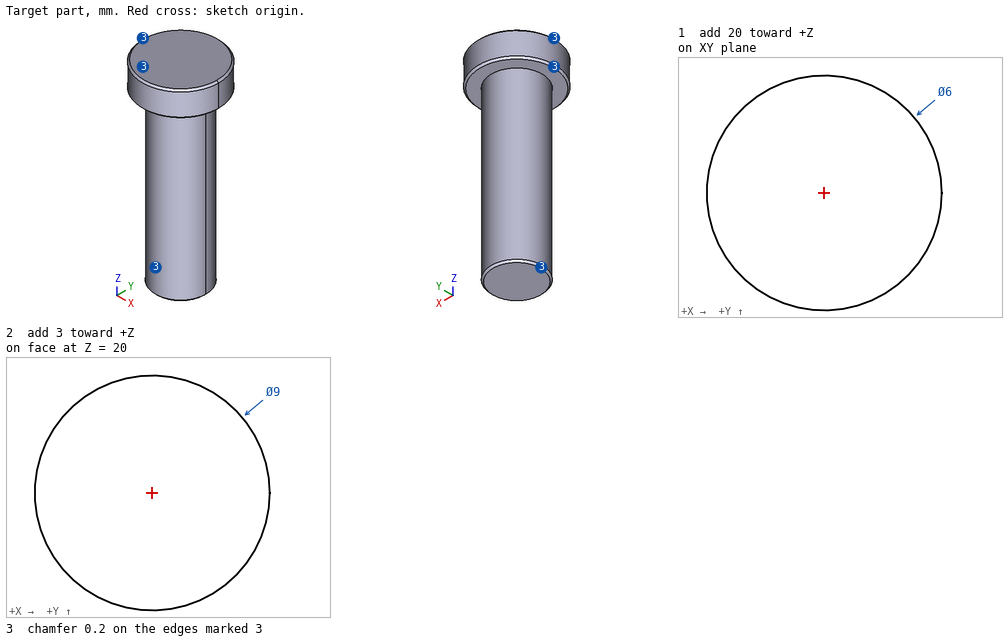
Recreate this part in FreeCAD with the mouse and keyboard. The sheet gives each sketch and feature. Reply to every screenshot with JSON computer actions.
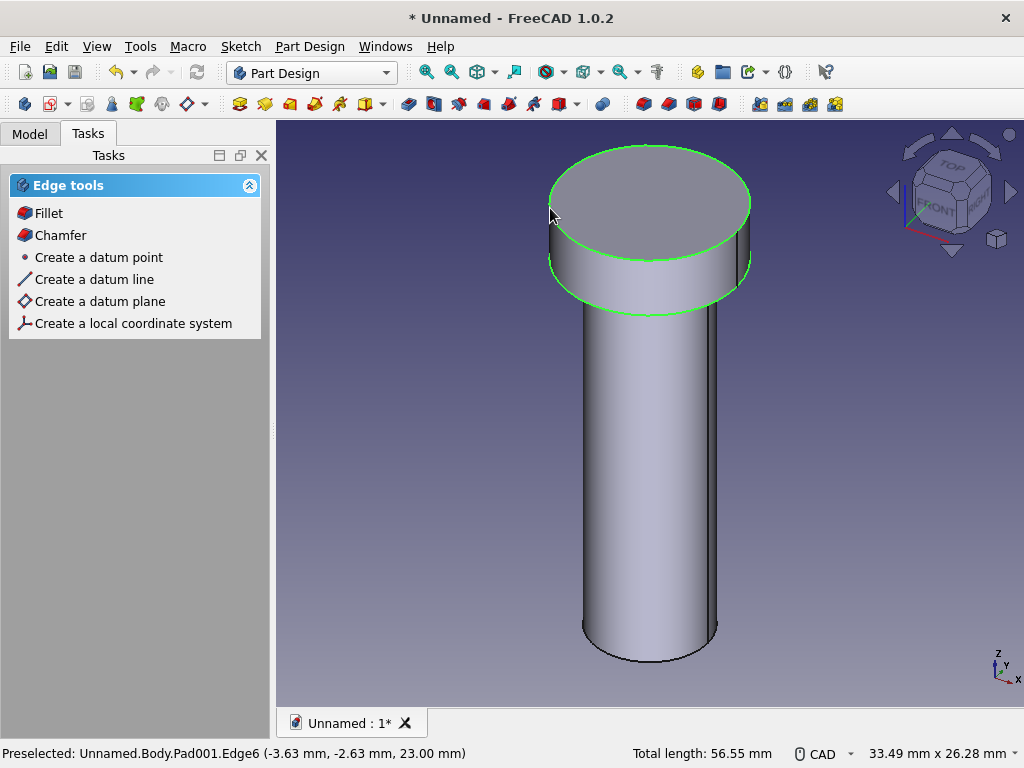
{"action": "key", "text": "0"}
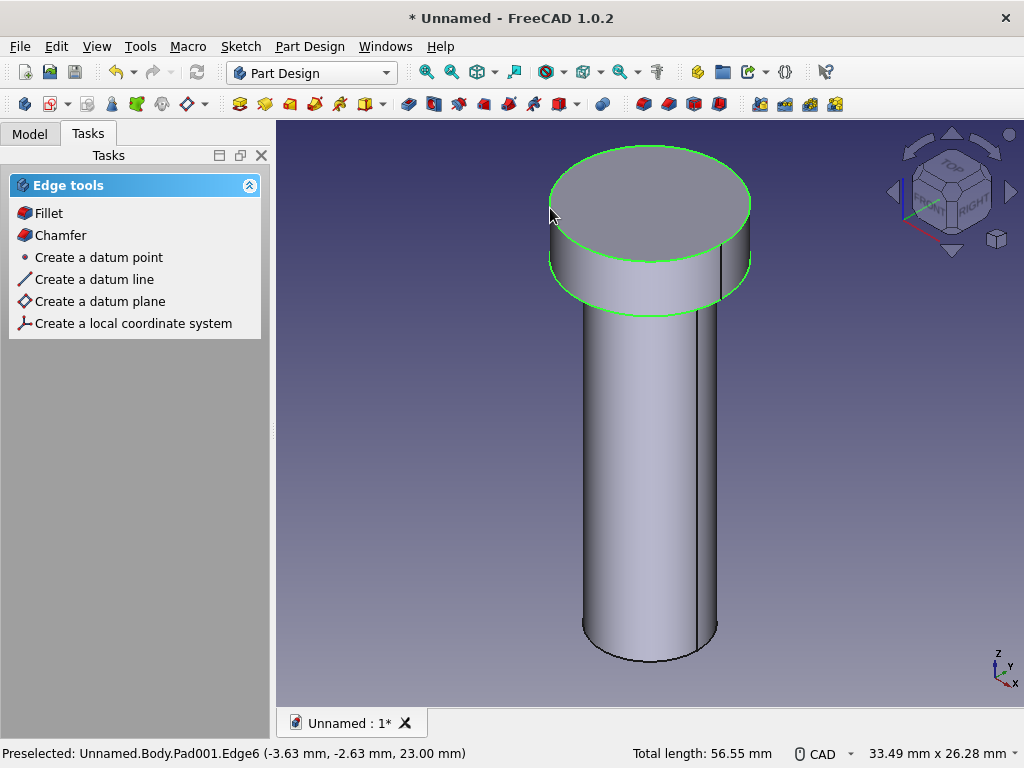
{"action": "key", "text": "2"}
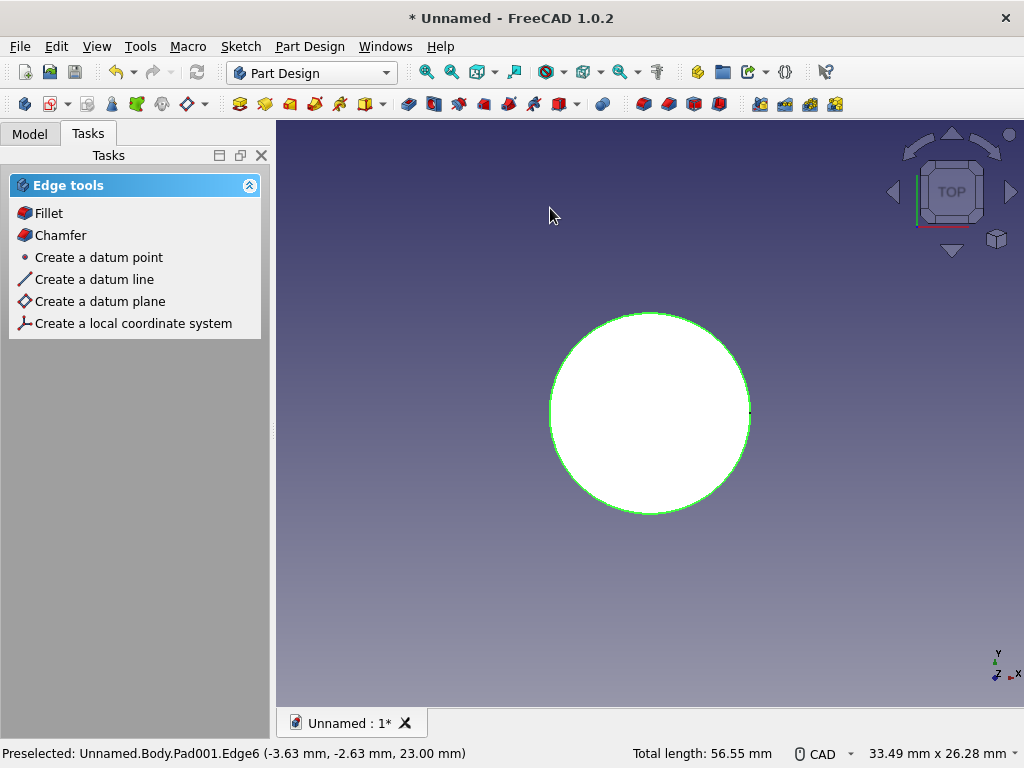
{"action": "left_click", "coordinate": [427, 72]}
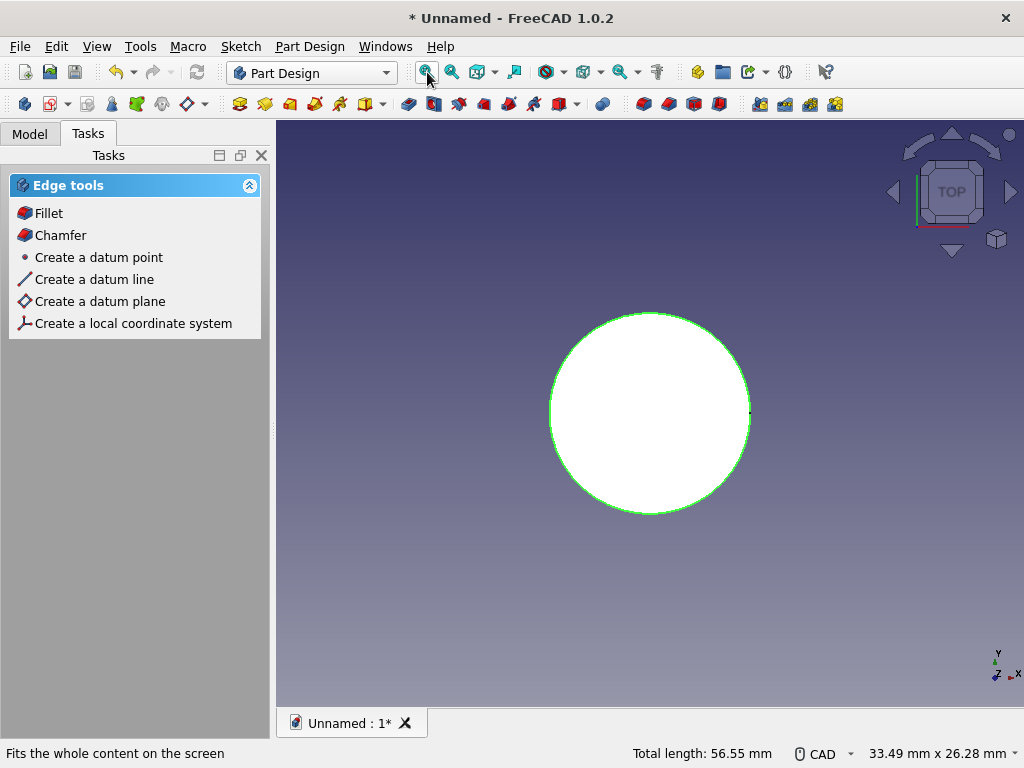
{"action": "key", "text": "1"}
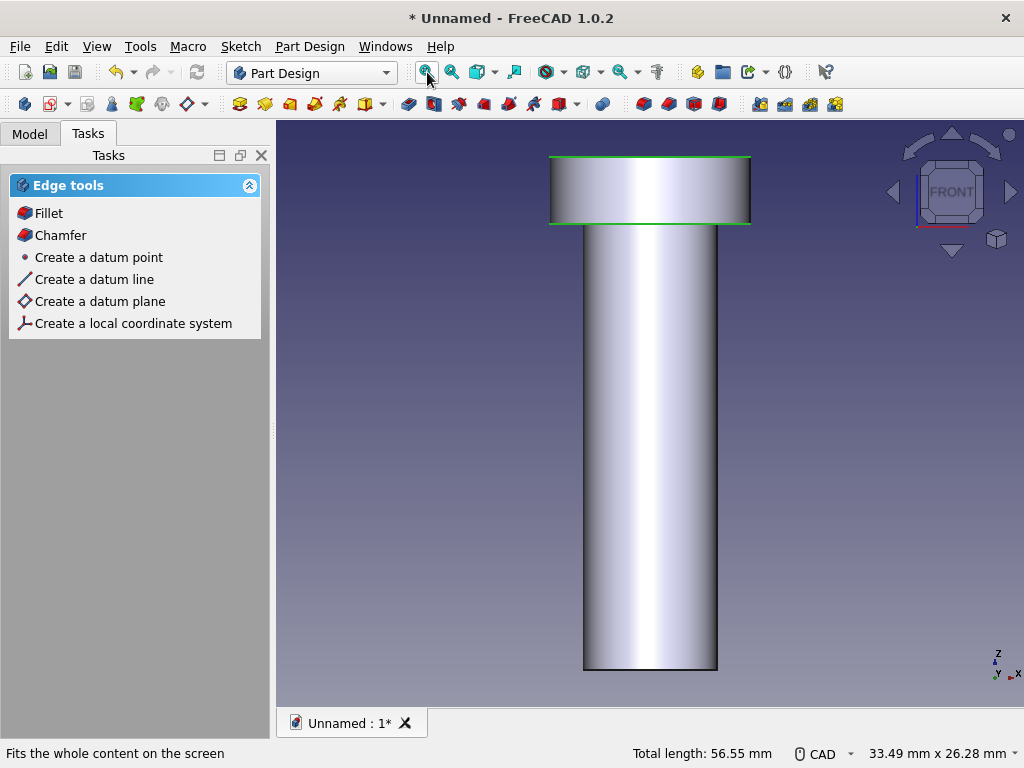
{"action": "left_click", "coordinate": [596, 669], "text": "ctrl"}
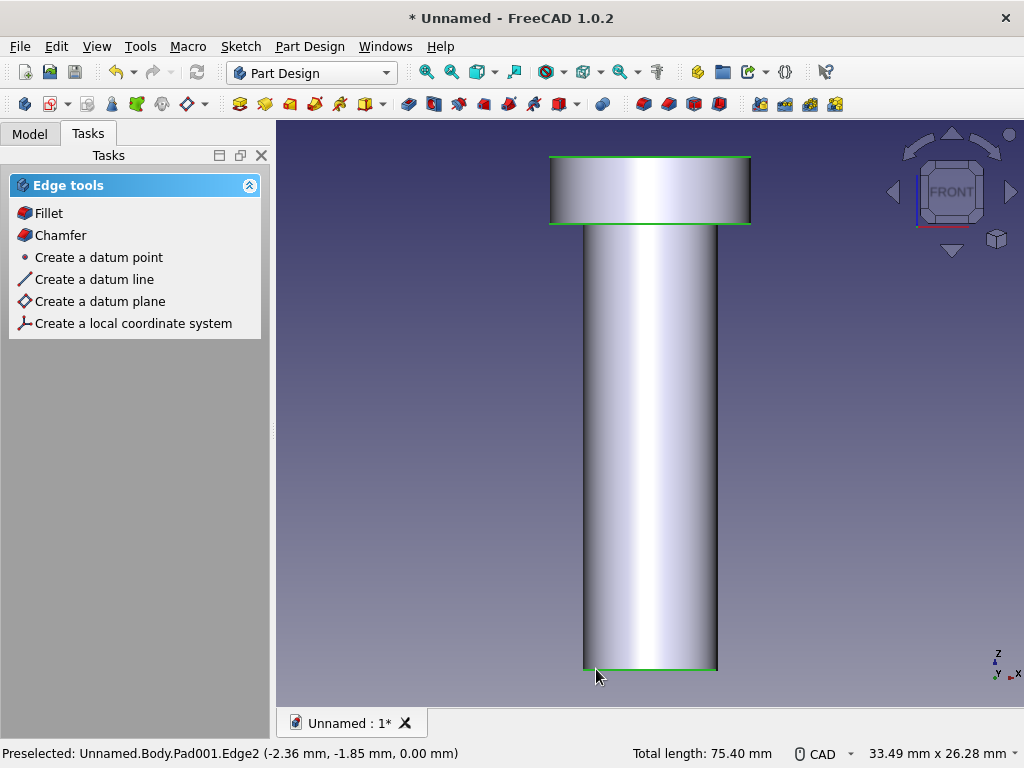
{"action": "left_click", "coordinate": [669, 104]}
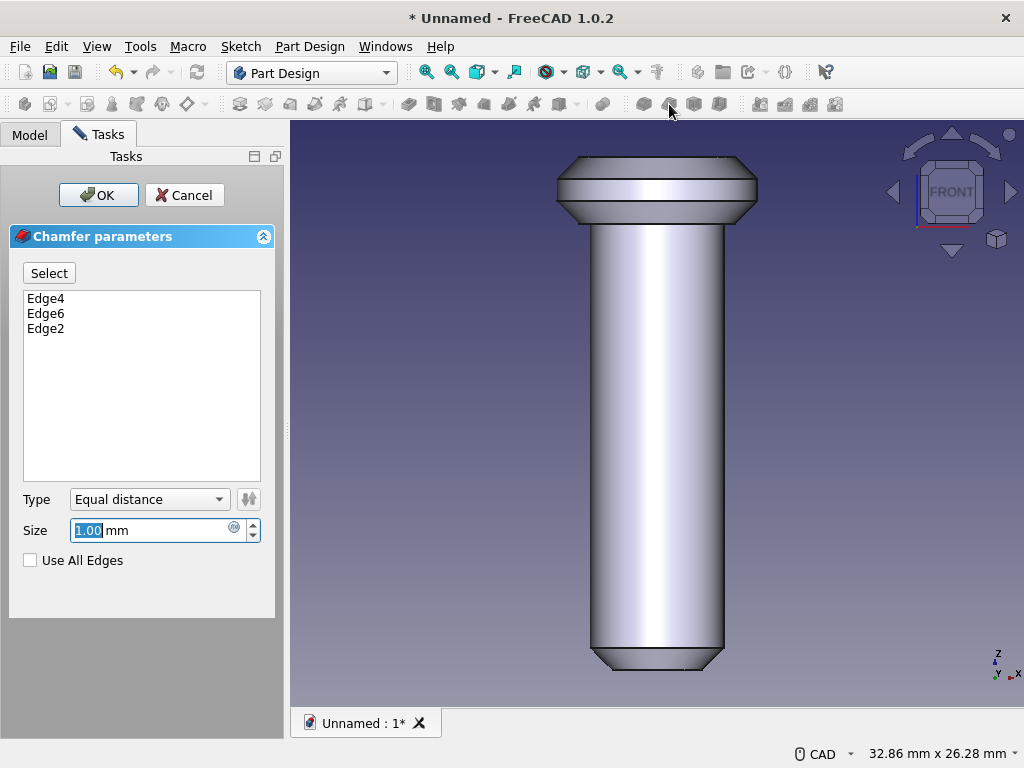
{"action": "type", "text": "0.2"}
{"action": "key", "text": "Tab"}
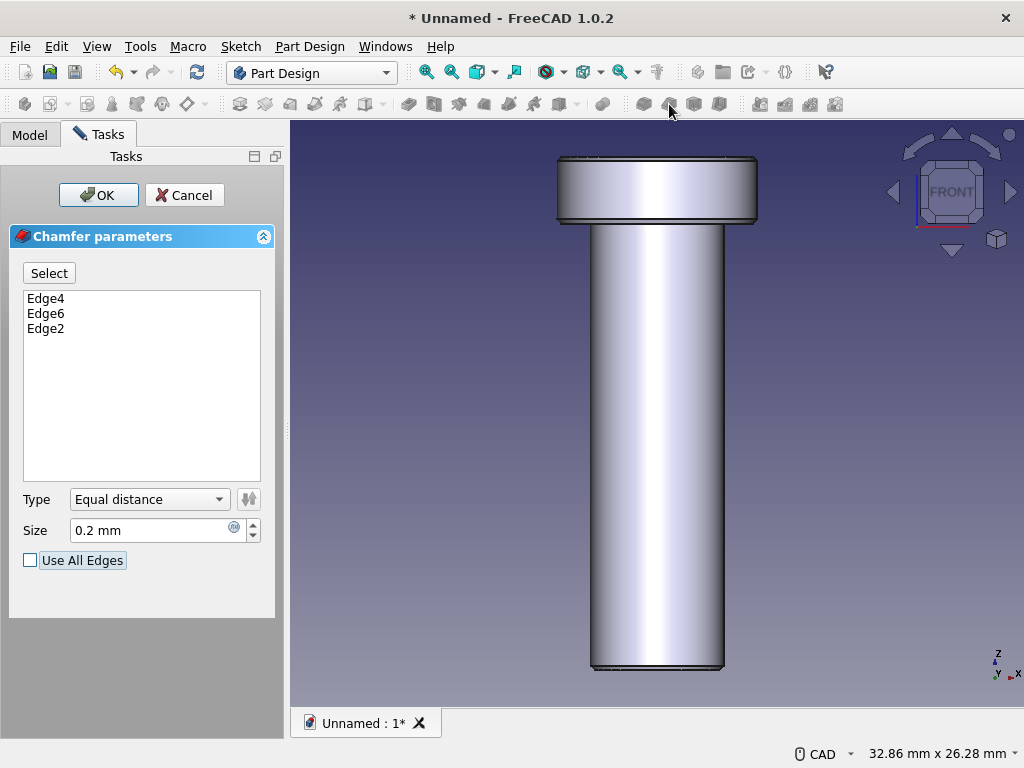
{"action": "left_click", "coordinate": [99, 195]}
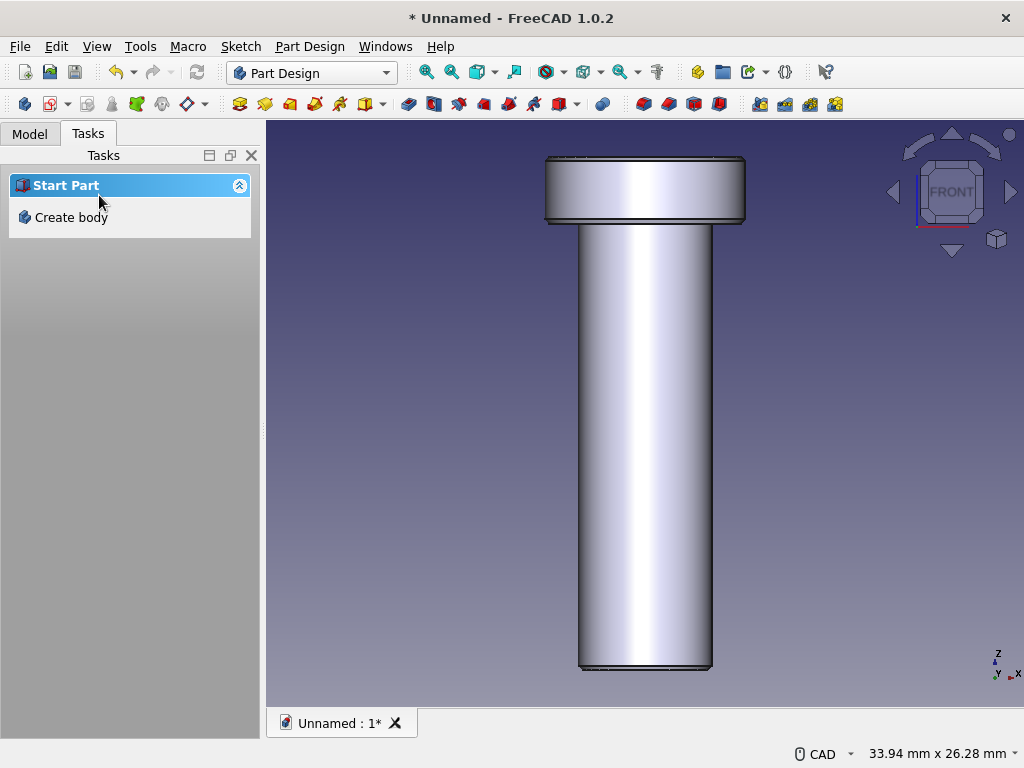
{"action": "key", "text": "0"}